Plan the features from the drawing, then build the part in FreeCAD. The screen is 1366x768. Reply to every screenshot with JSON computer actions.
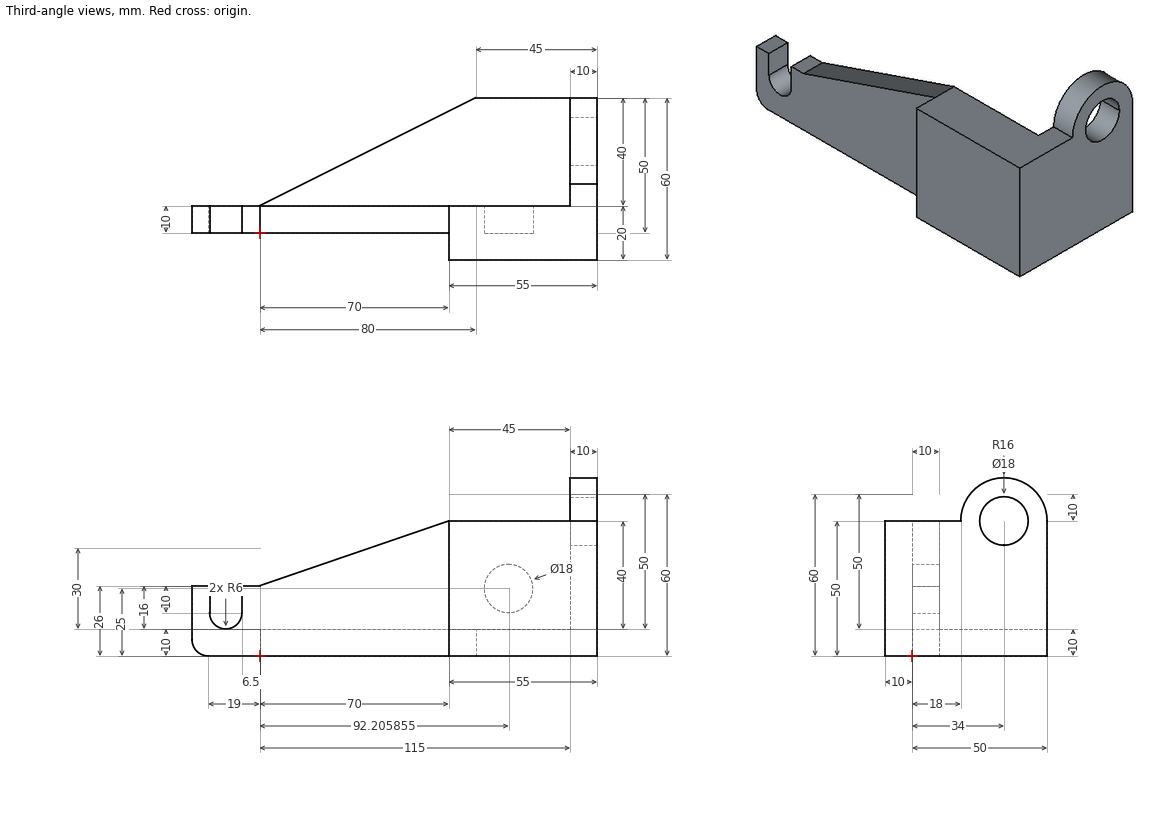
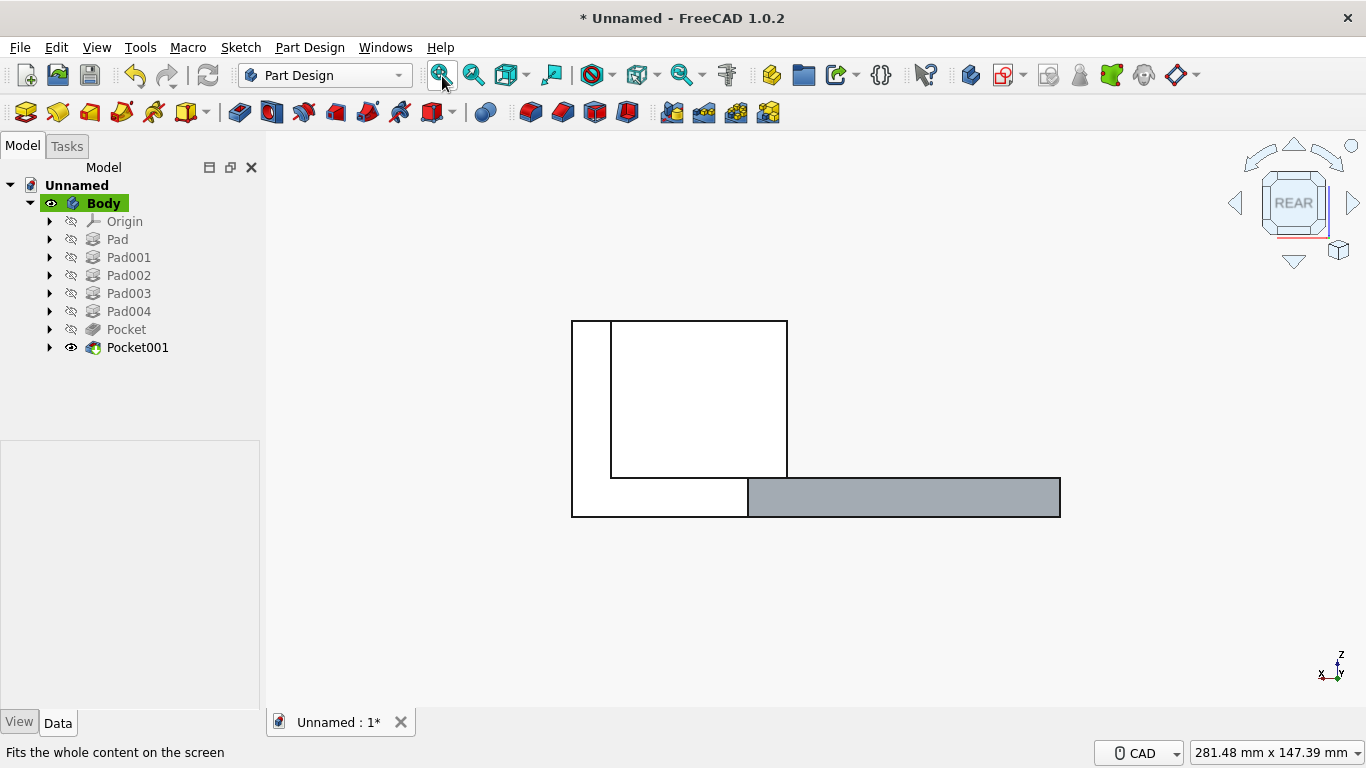
{"action": "left_click", "coordinate": [699, 398]}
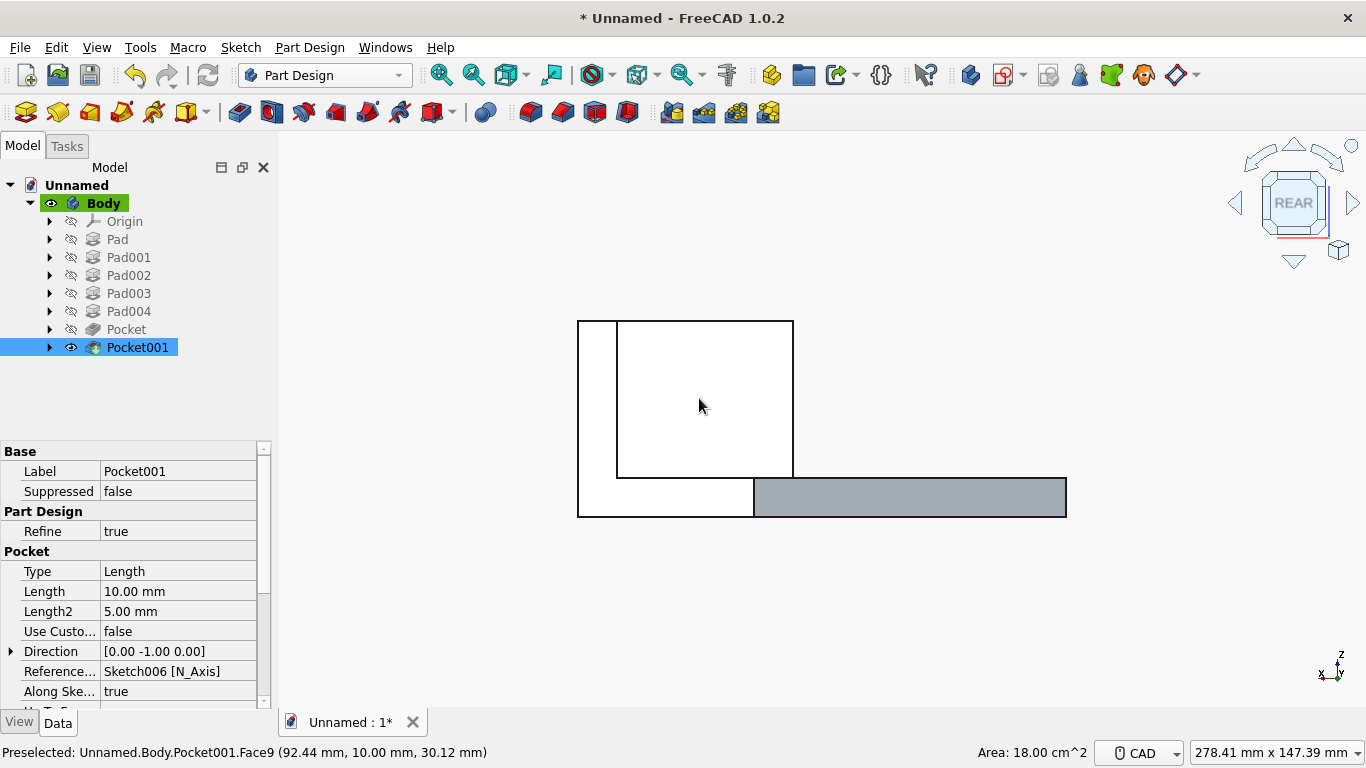
{"action": "left_click", "coordinate": [1004, 76]}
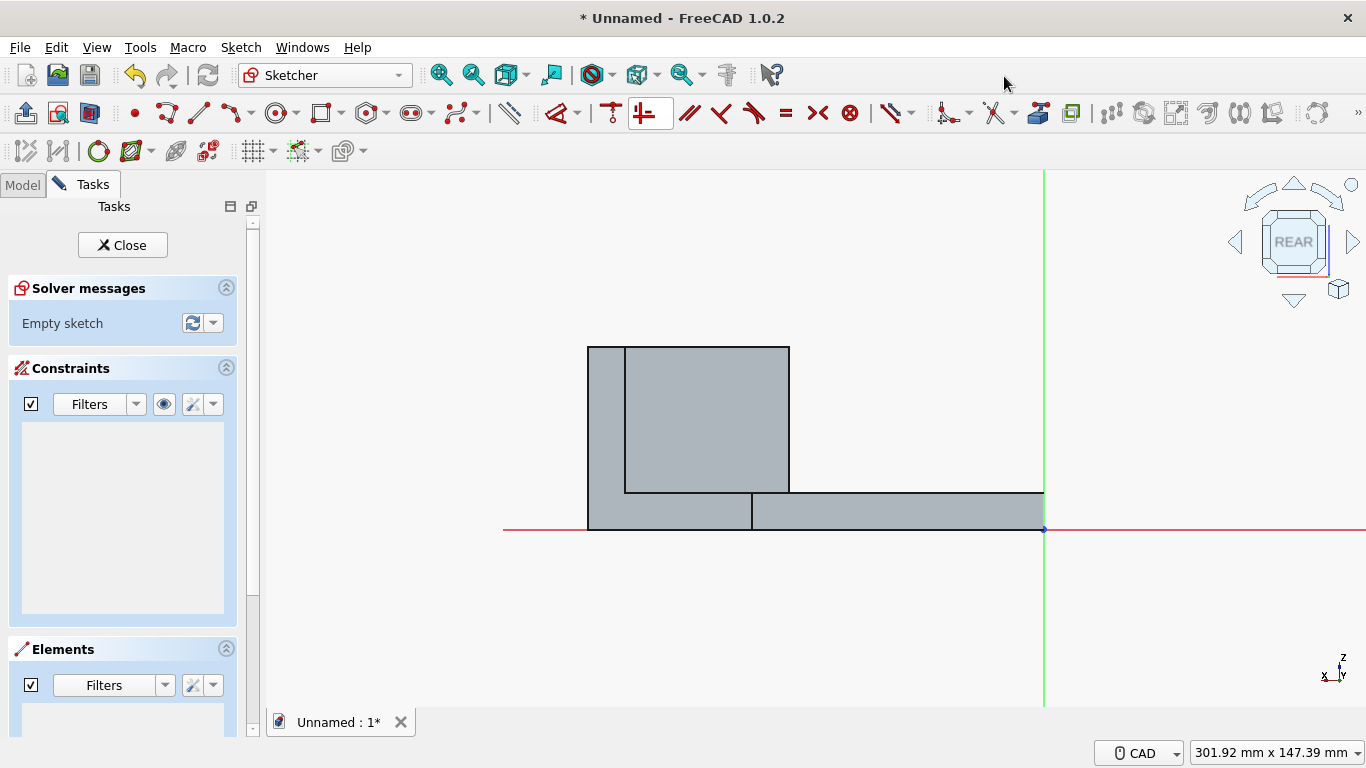
{"action": "scroll", "coordinate": [1121, 439], "scroll_direction": "up", "scroll_amount": 3}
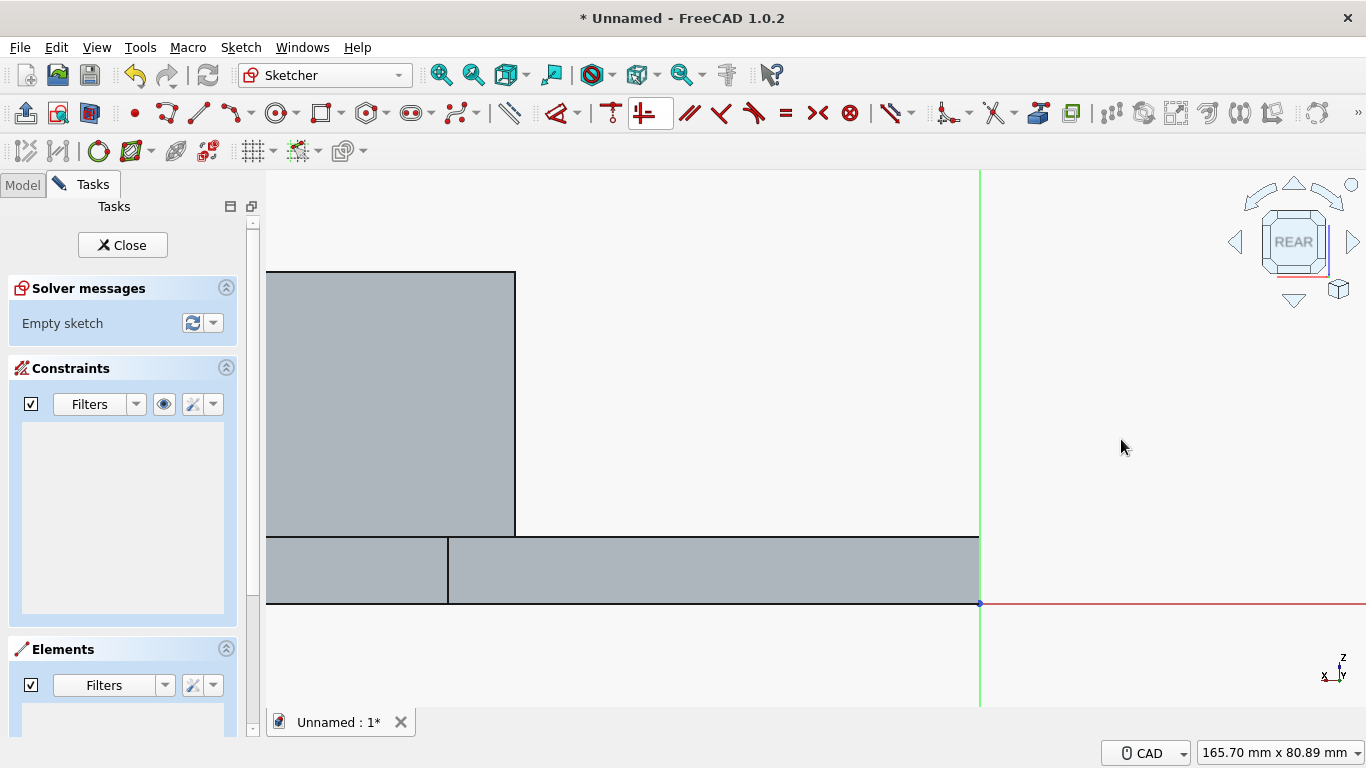
{"action": "left_click", "coordinate": [168, 114]}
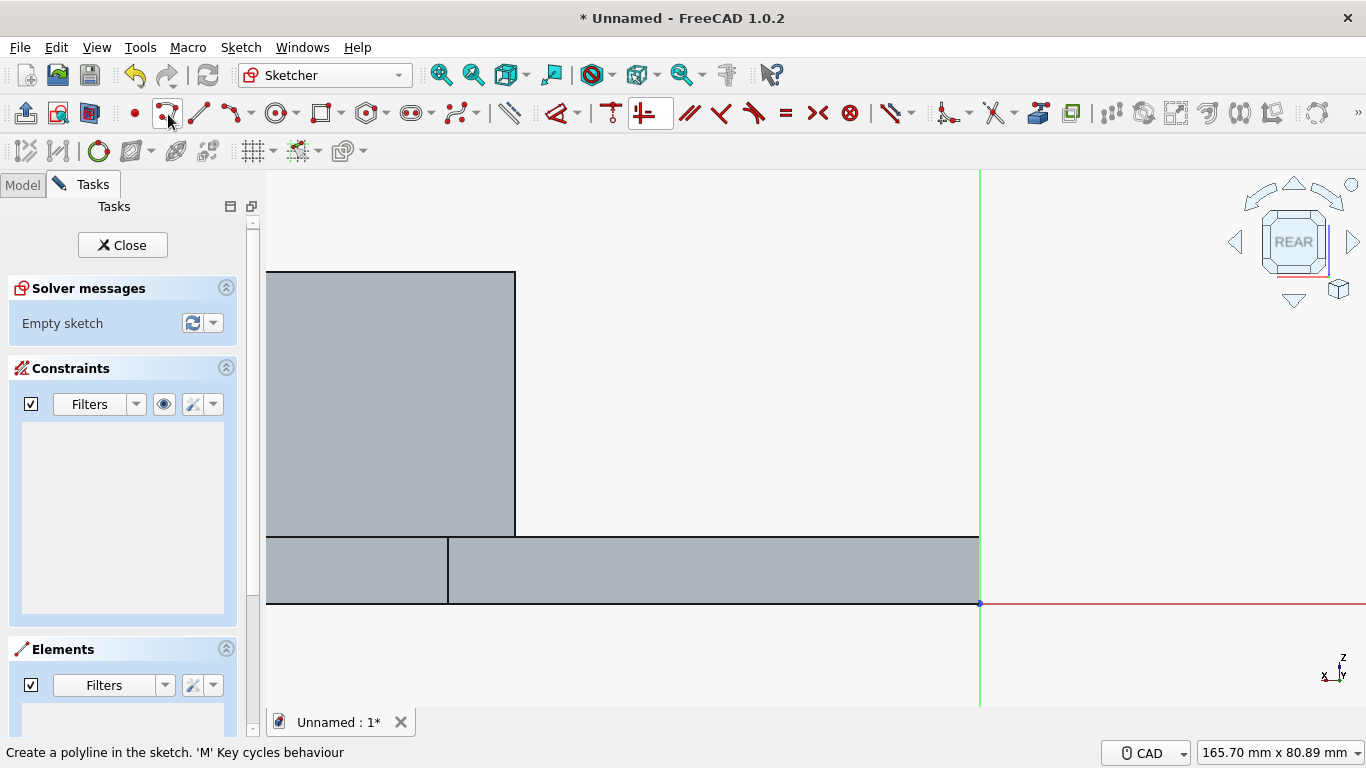
{"action": "left_click", "coordinate": [980, 537]}
{"action": "left_click", "coordinate": [971, 431]}
{"action": "left_click", "coordinate": [515, 272]}
{"action": "left_click", "coordinate": [515, 537]}
{"action": "left_click", "coordinate": [980, 538]}
{"action": "key", "text": "Escape"}
{"action": "key", "text": "Escape"}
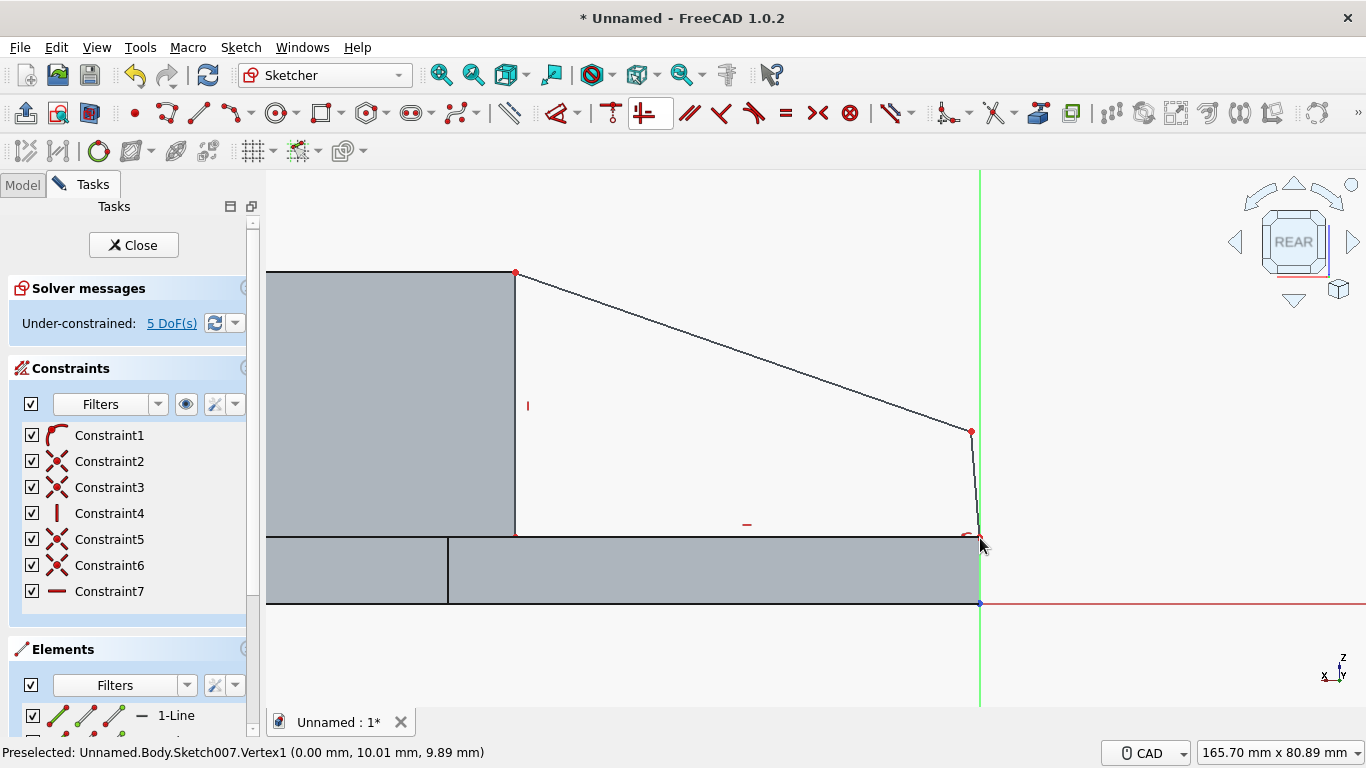
{"action": "left_click", "coordinate": [977, 506]}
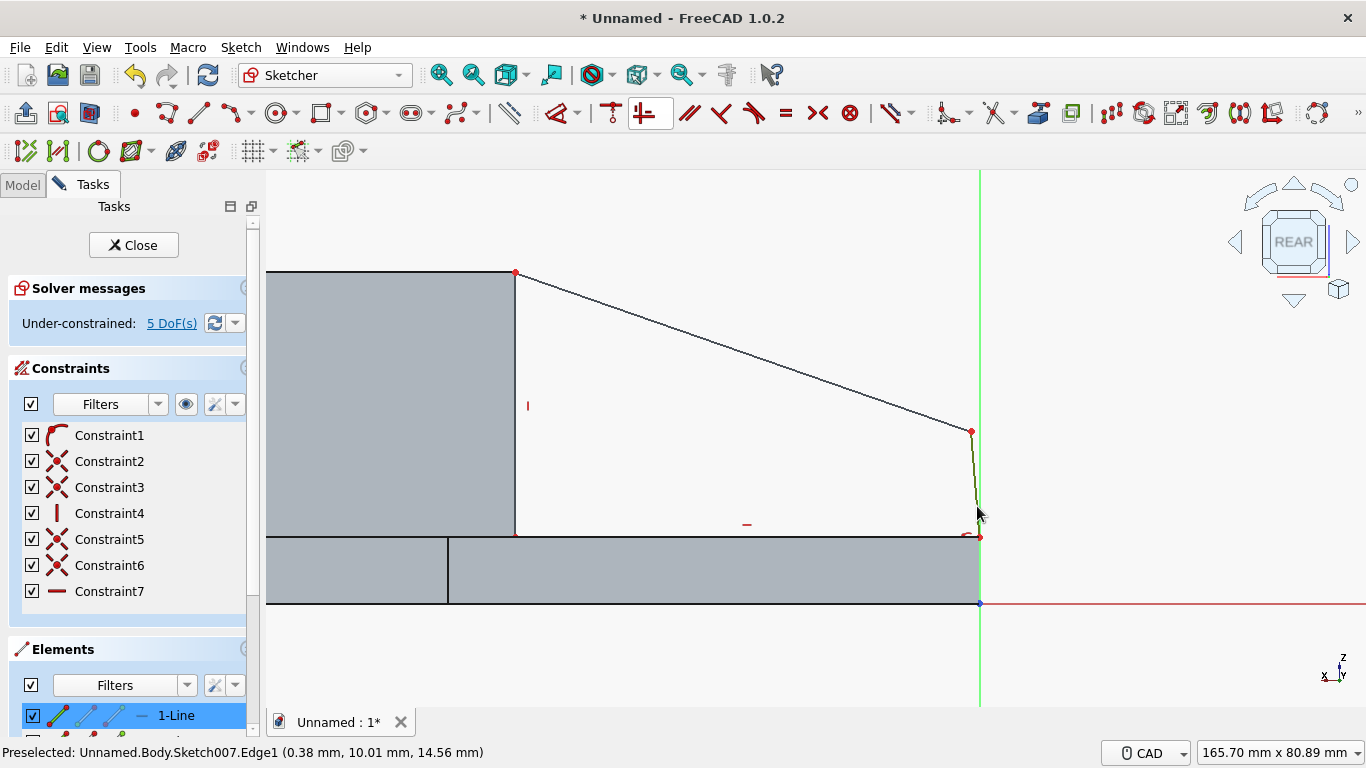
{"action": "left_click", "coordinate": [668, 114]}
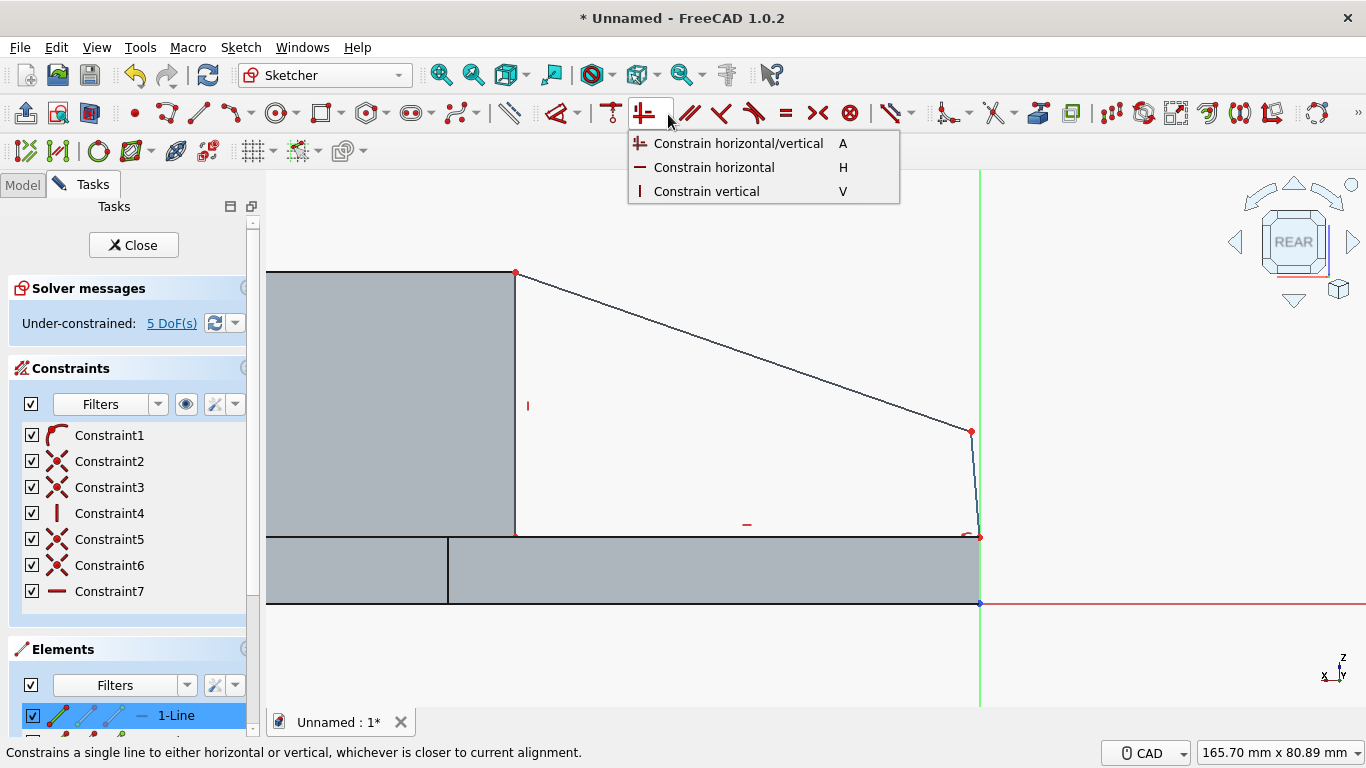
{"action": "left_click", "coordinate": [764, 191]}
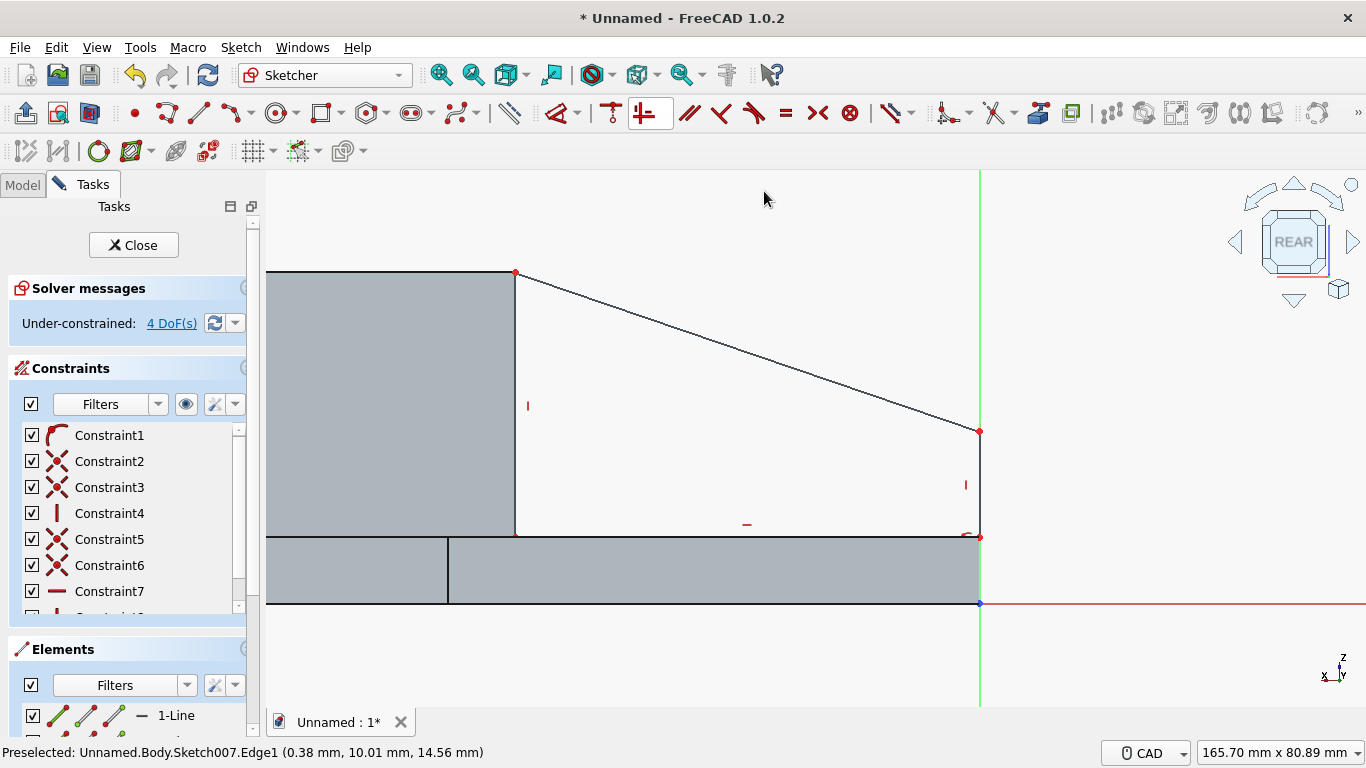
{"action": "left_click", "coordinate": [556, 114]}